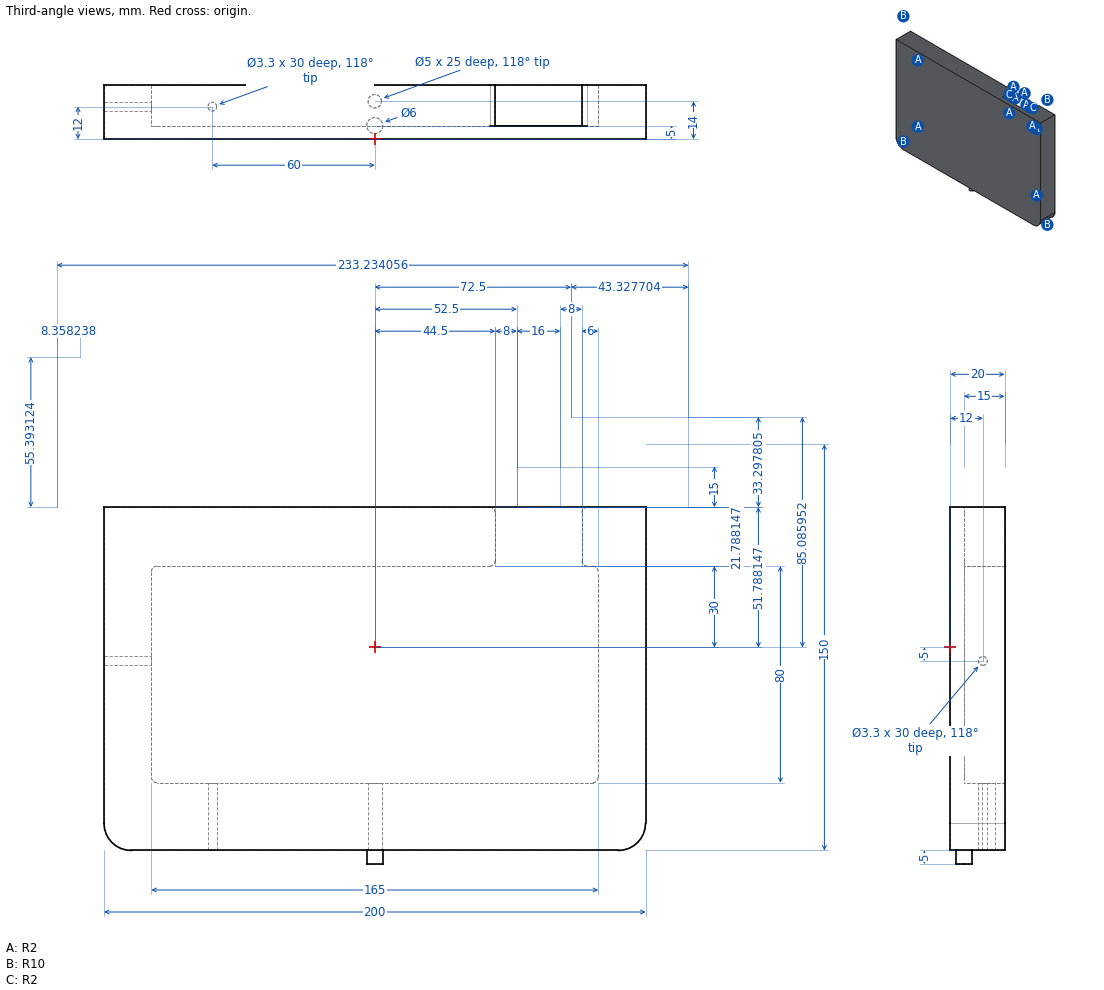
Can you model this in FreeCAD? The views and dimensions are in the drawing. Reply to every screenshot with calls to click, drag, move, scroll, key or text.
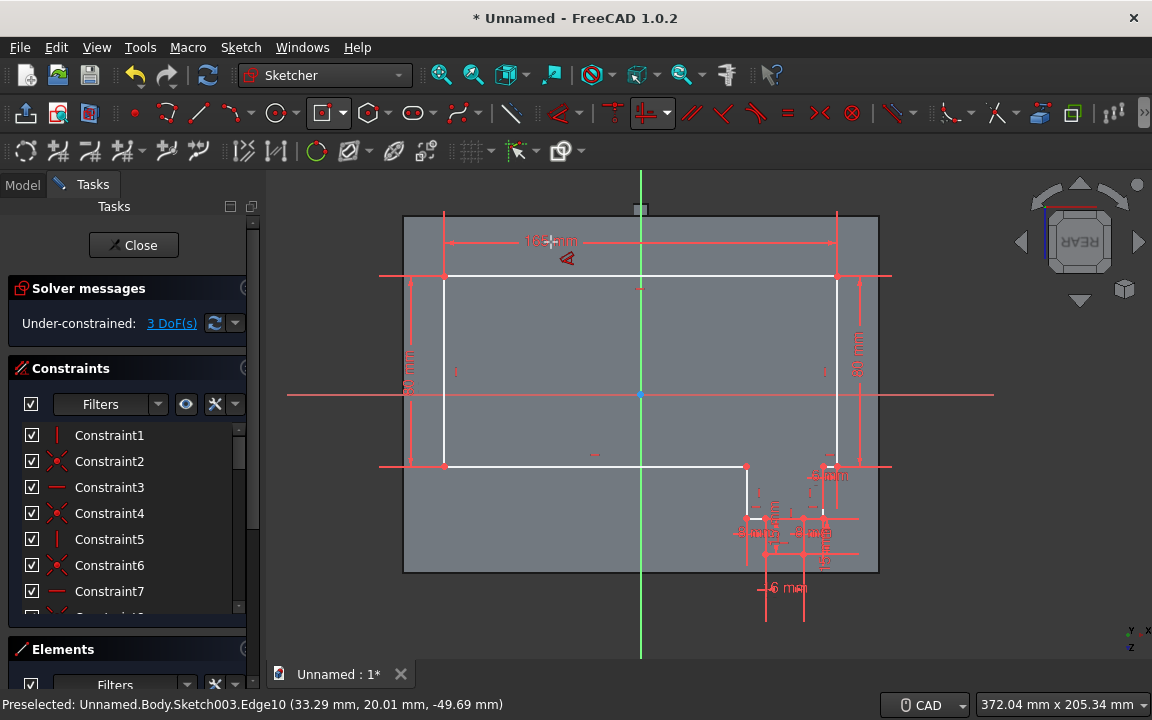
click(747, 467)
click(781, 431)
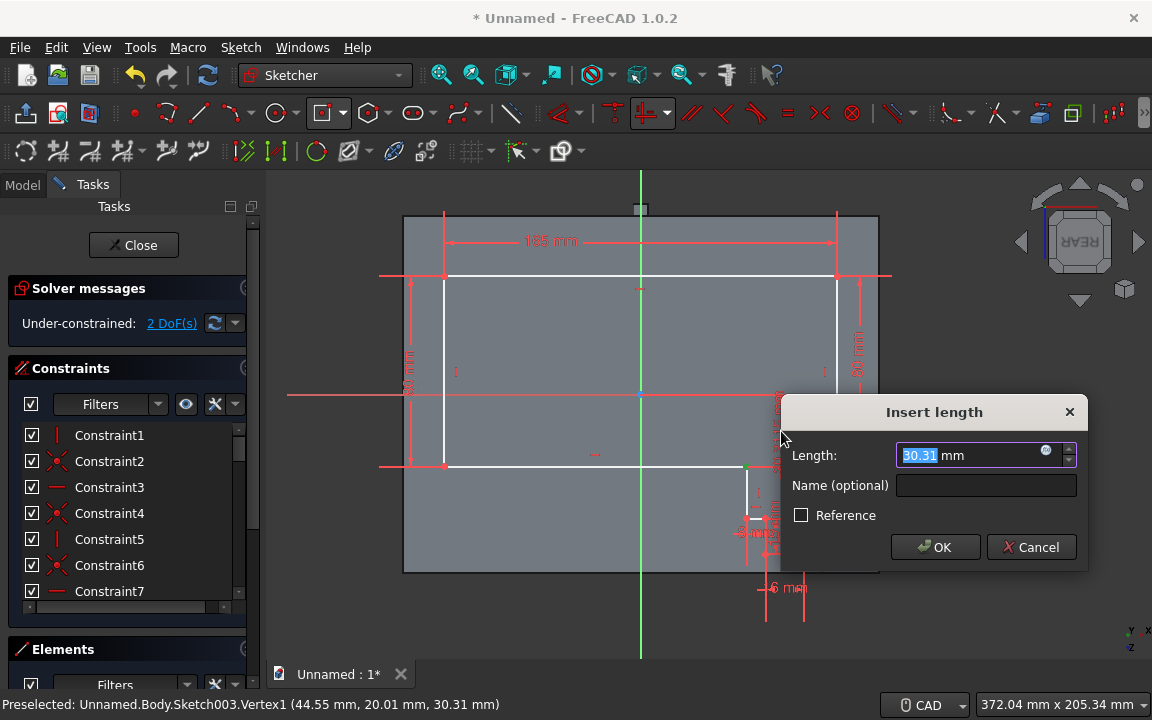
text(30)
key(Return)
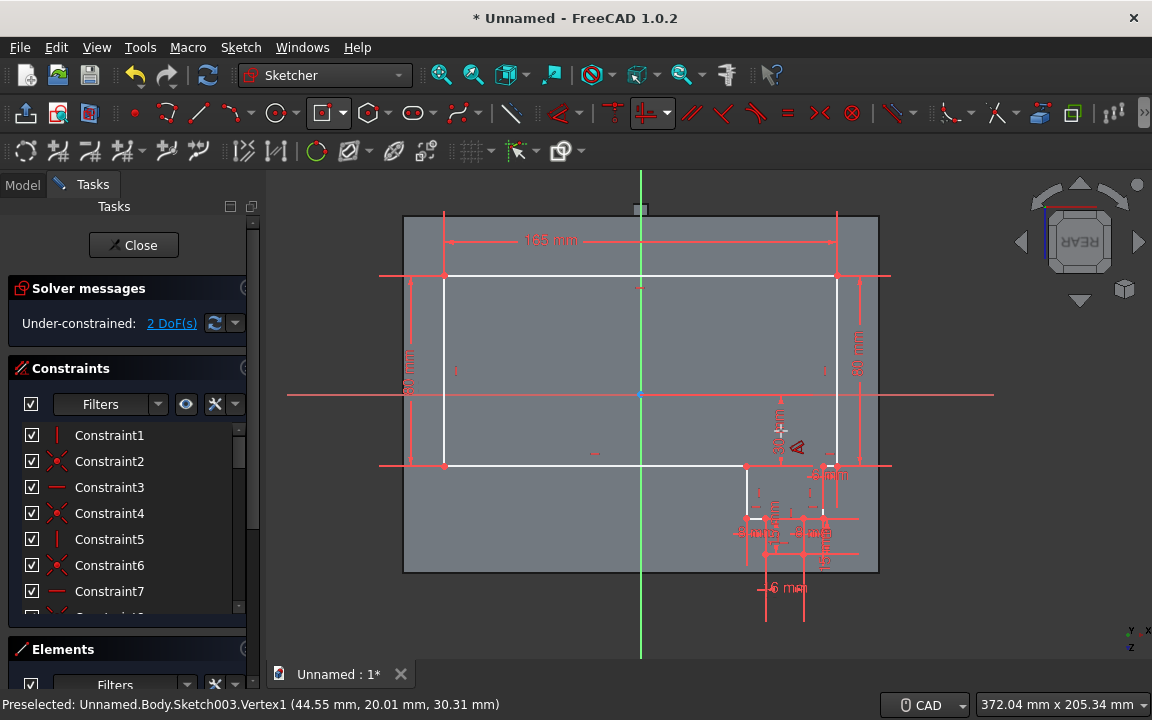
click(747, 466)
click(694, 500)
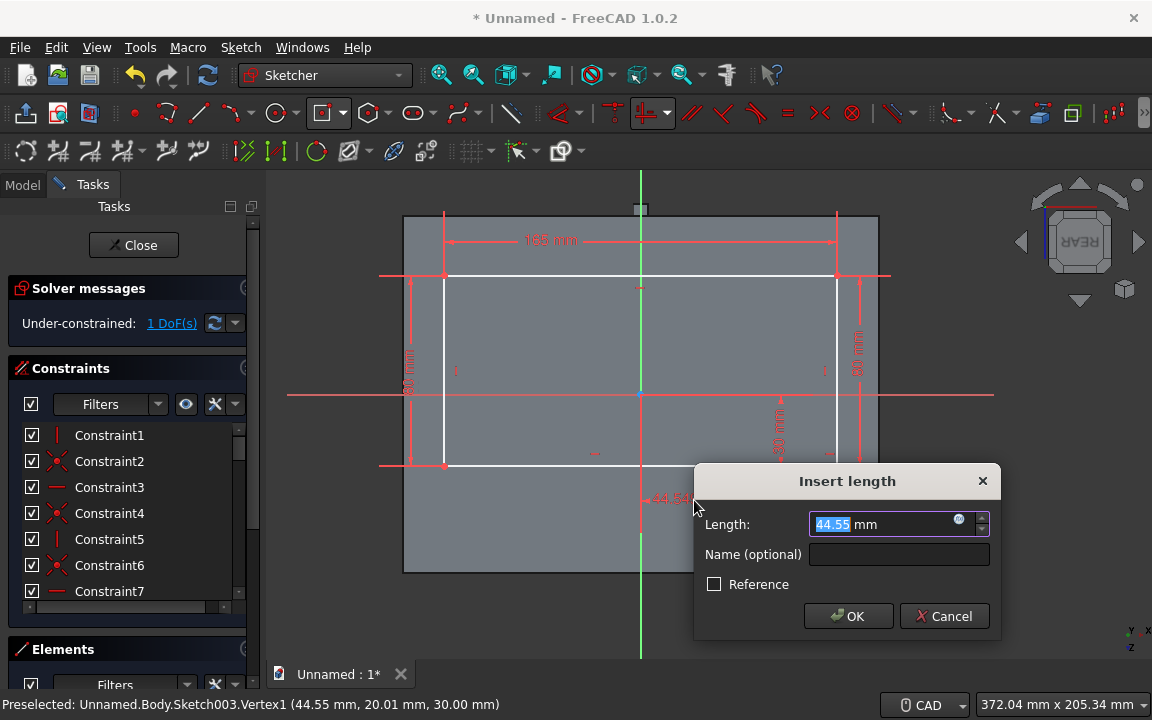
text(44.5)
key(Return)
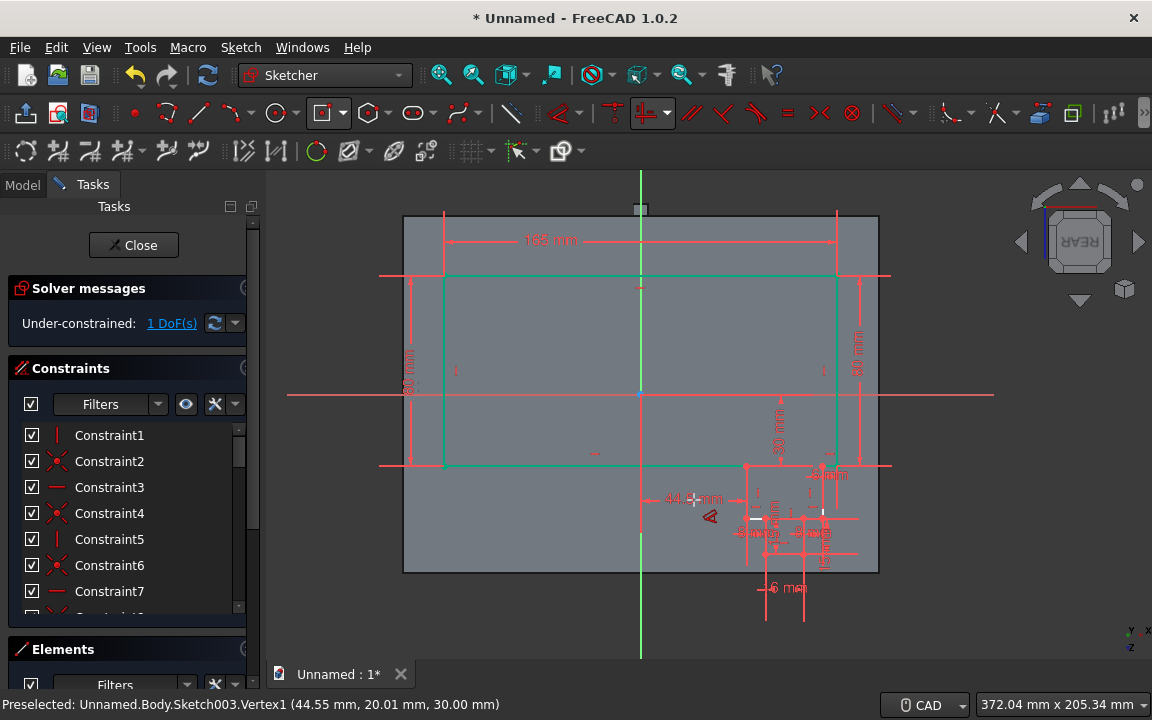
click(747, 482)
click(853, 504)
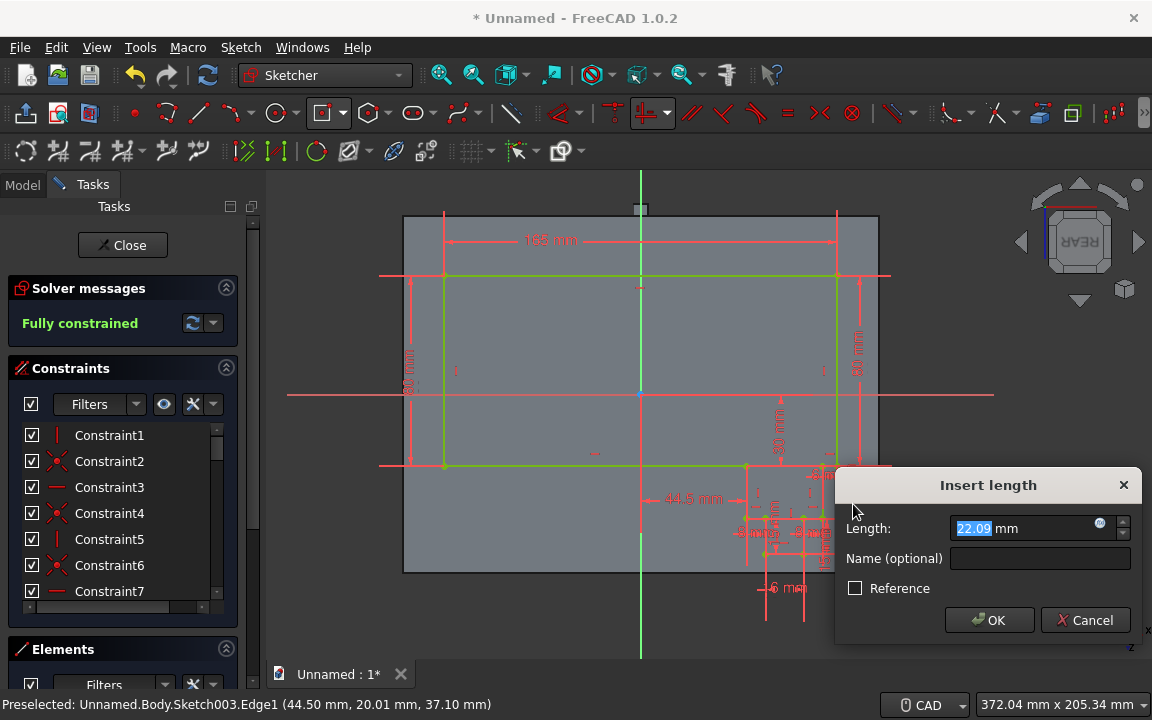
text(21.788147)
key(Return)
key(Escape)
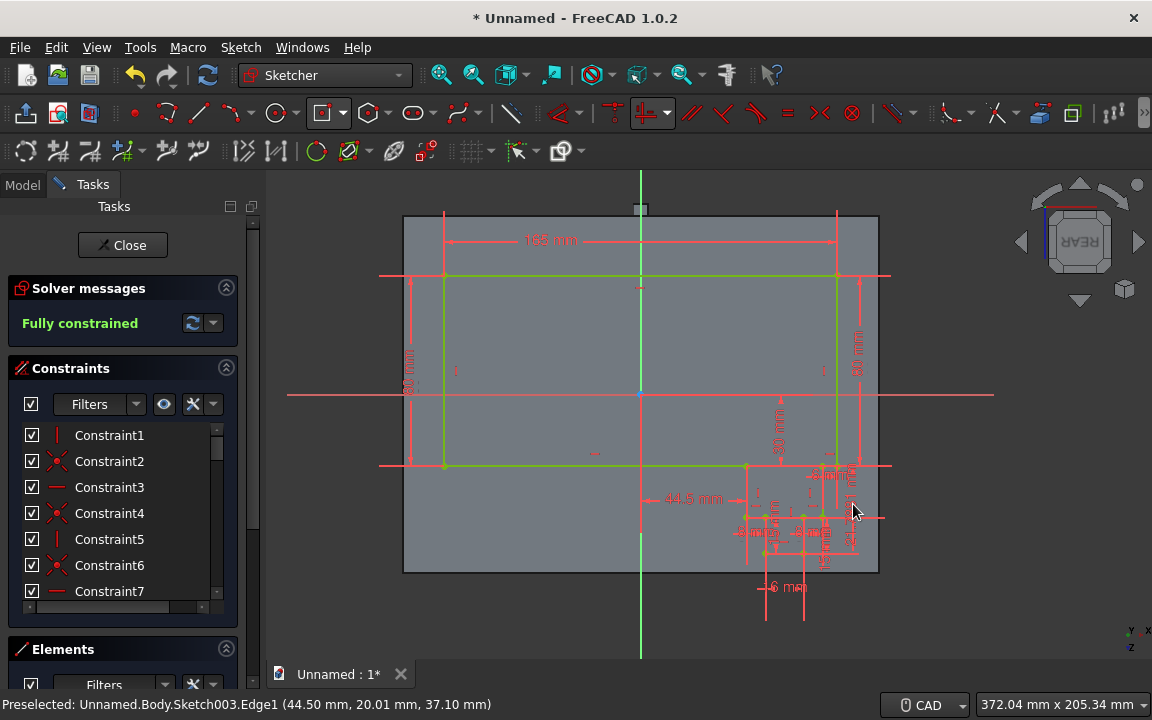
click(123, 245)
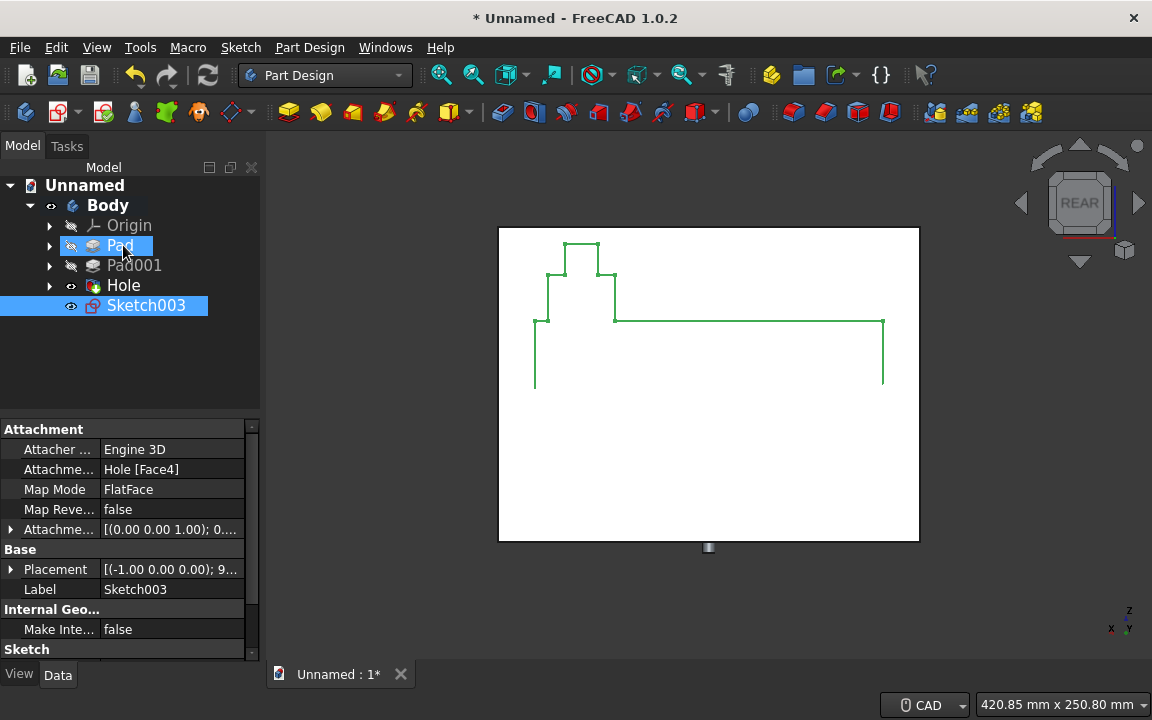
click(504, 112)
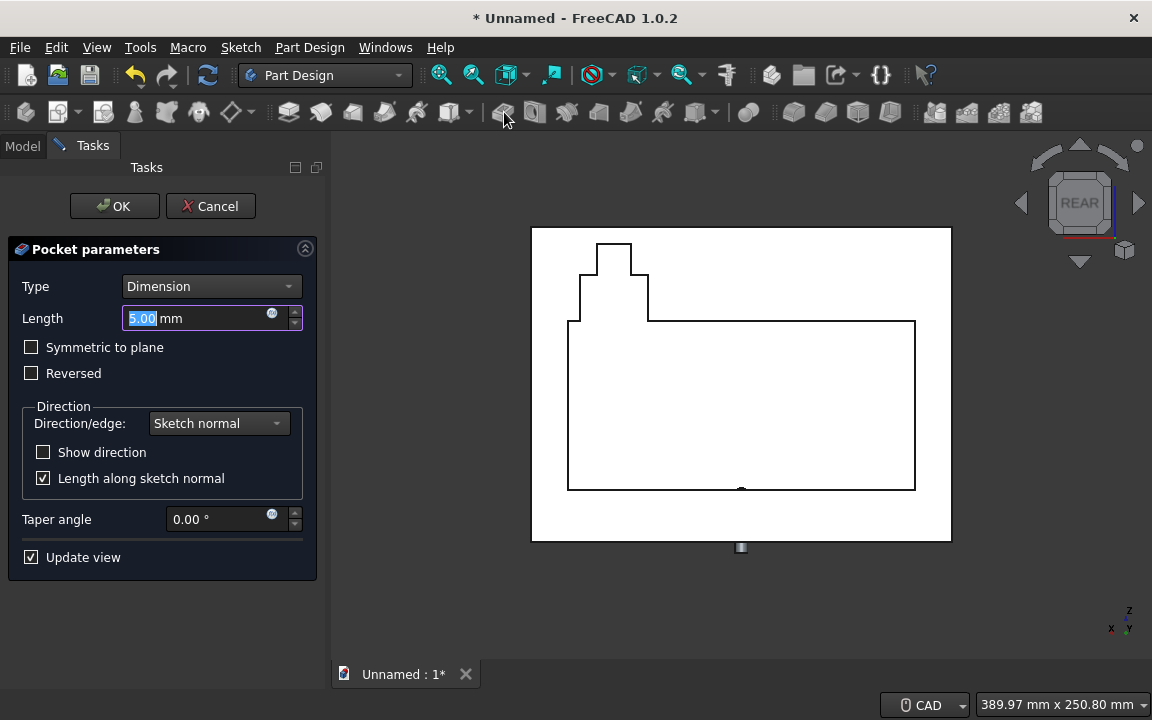
text(15)
key(Tab)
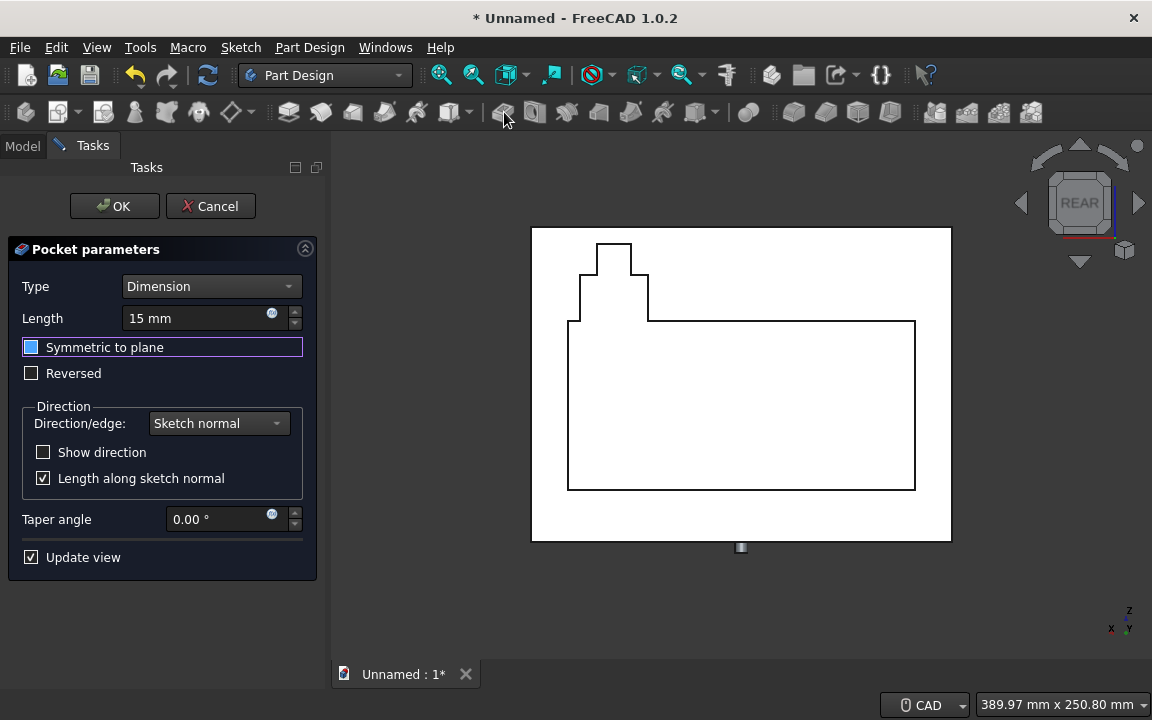
click(115, 206)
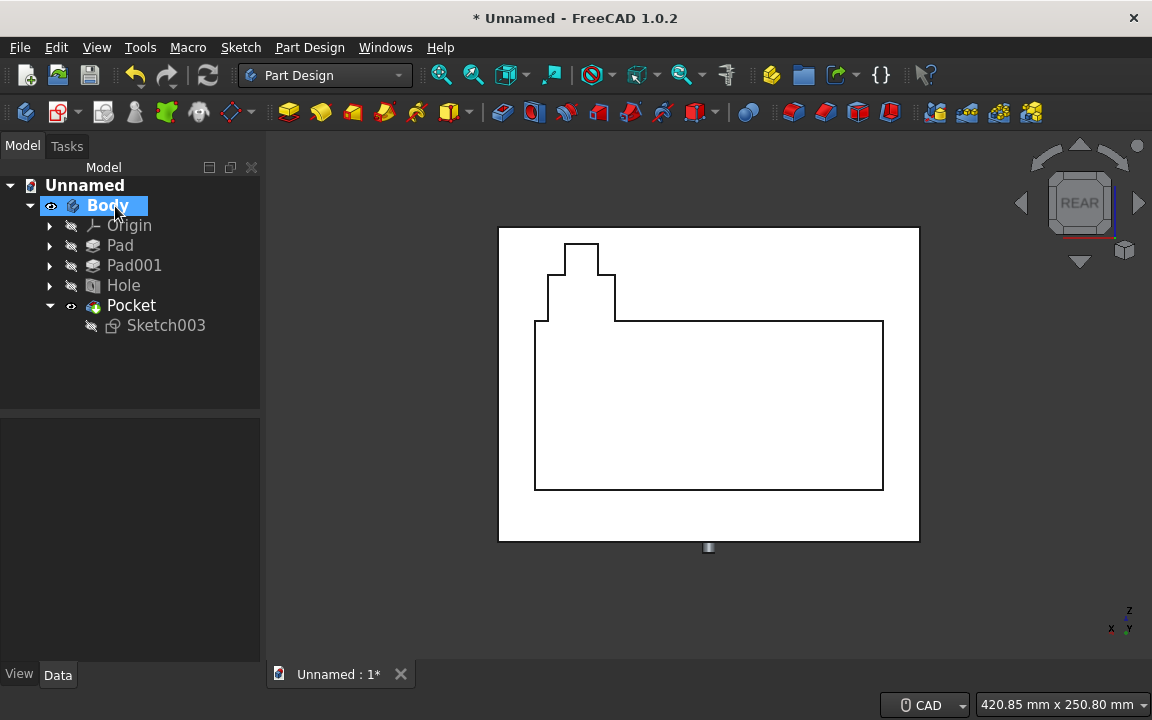
click(659, 401)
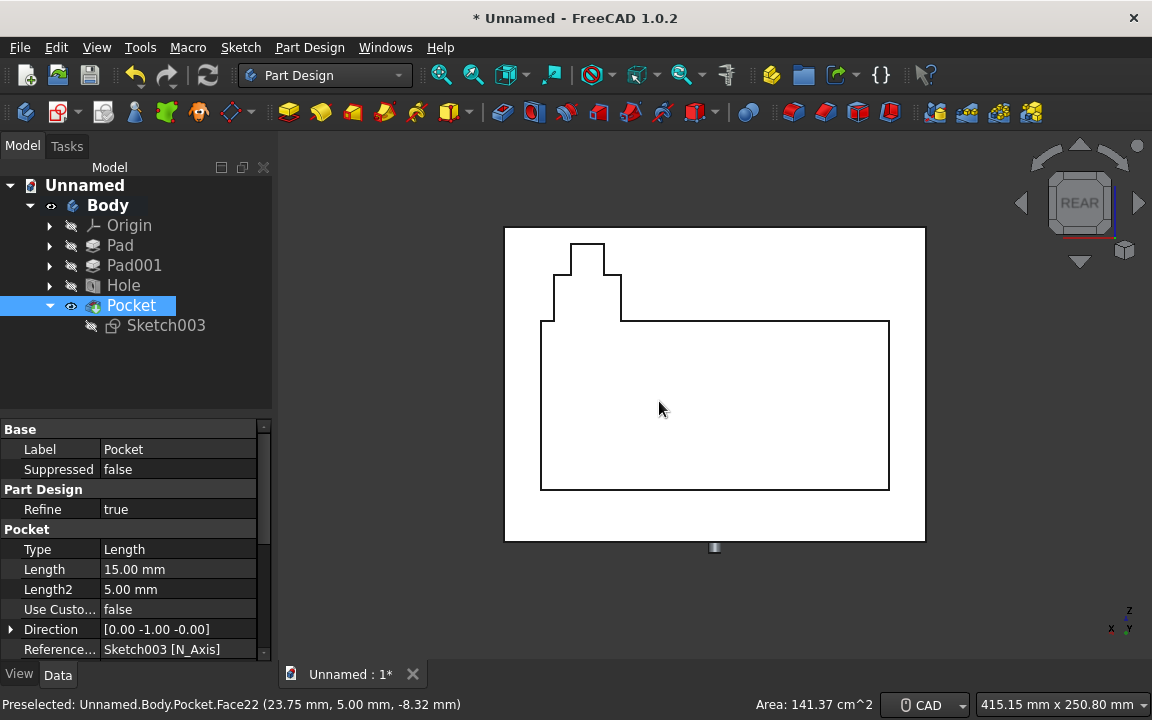
click(58, 112)